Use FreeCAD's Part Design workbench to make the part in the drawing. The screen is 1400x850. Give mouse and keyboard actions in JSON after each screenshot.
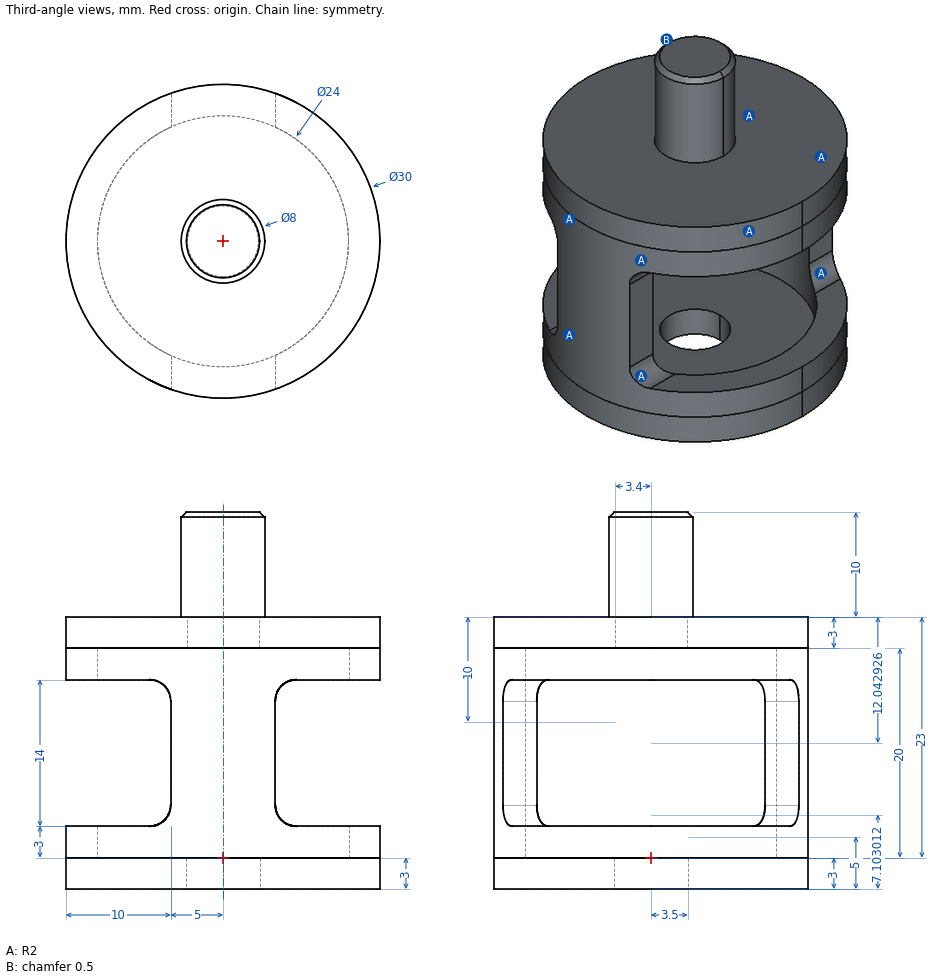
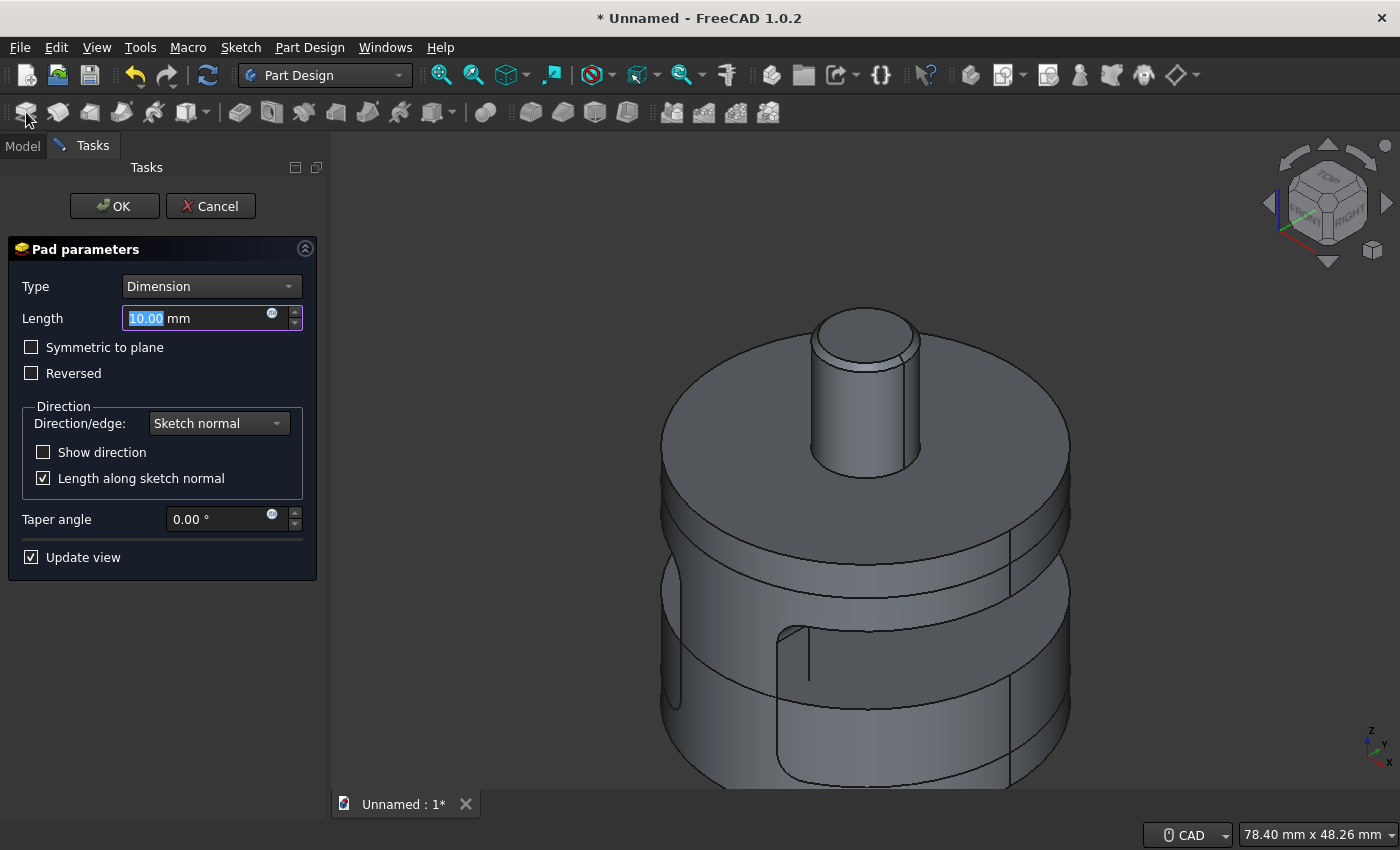
{"action": "type", "text": "3"}
{"action": "key", "text": "Tab"}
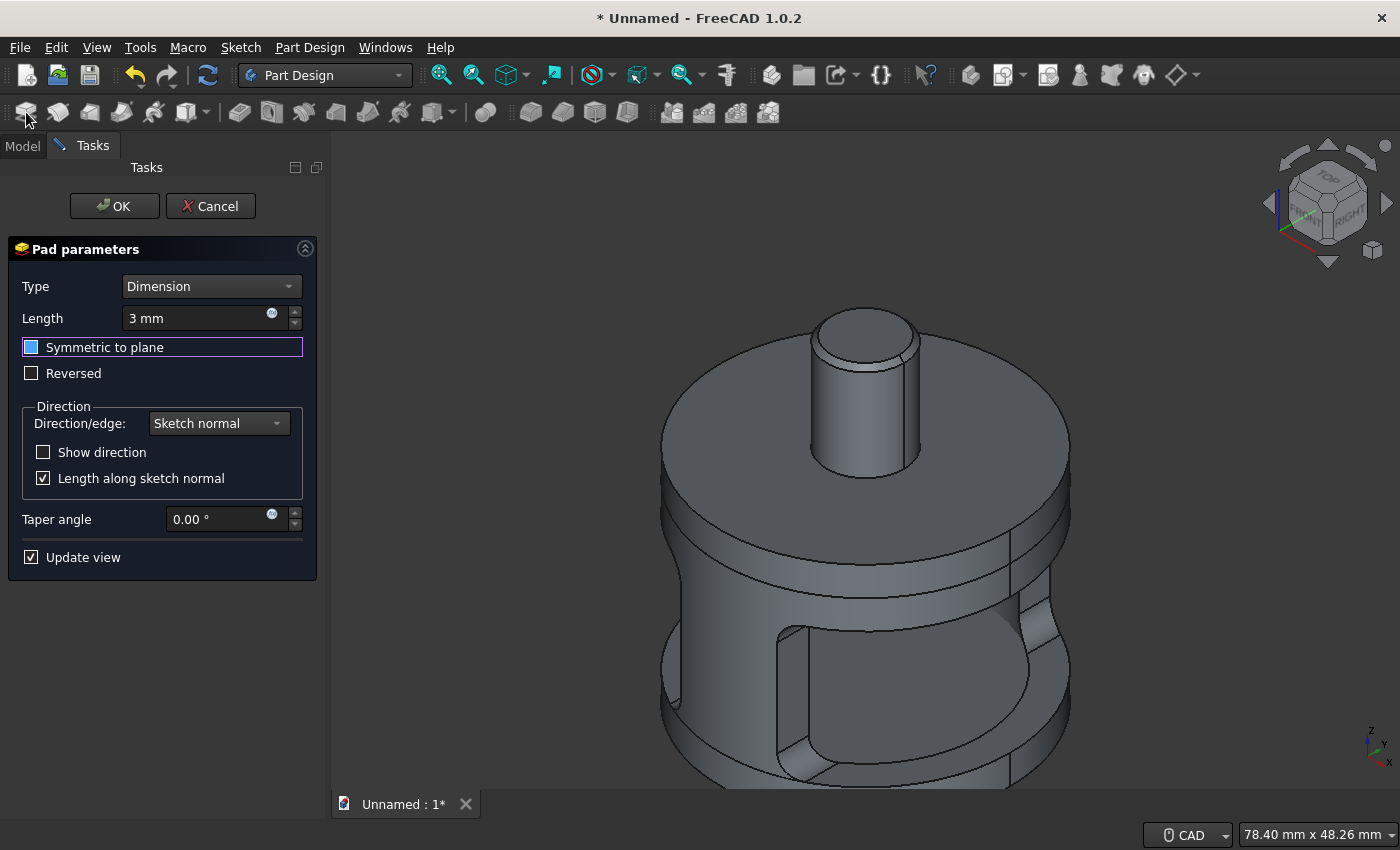
{"action": "left_click", "coordinate": [30, 373]}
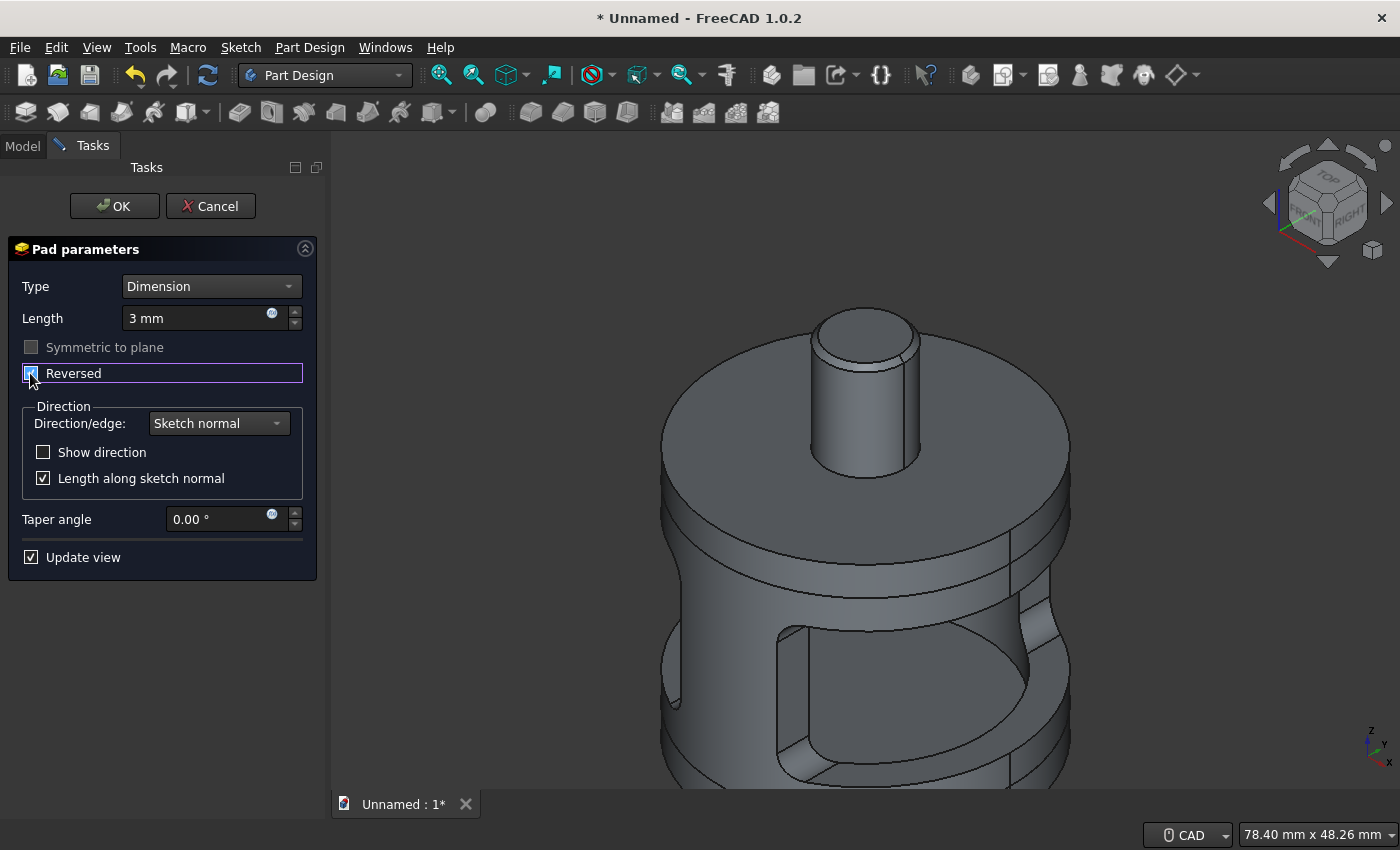
{"action": "left_click", "coordinate": [115, 206]}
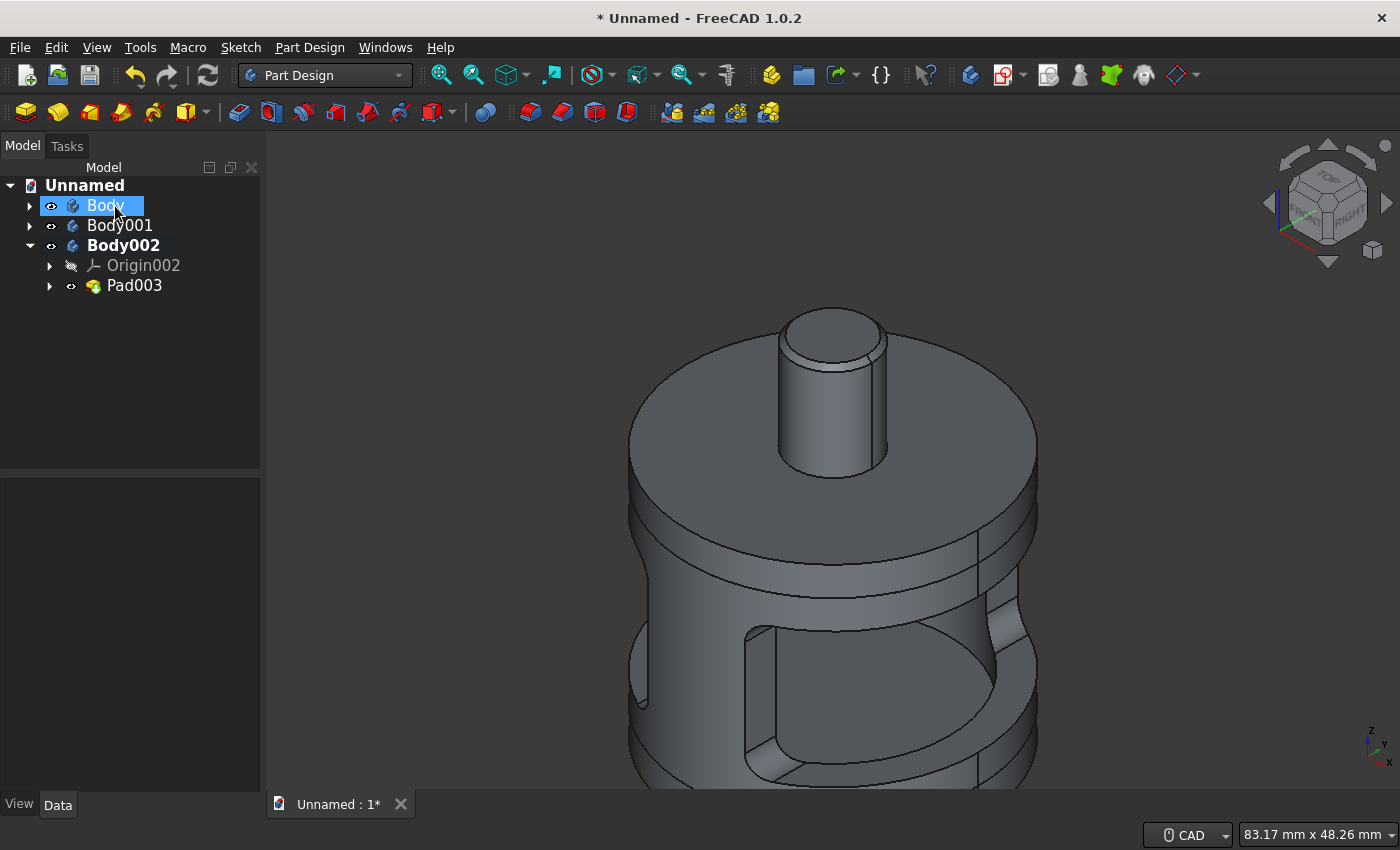
{"action": "left_click", "coordinate": [442, 76]}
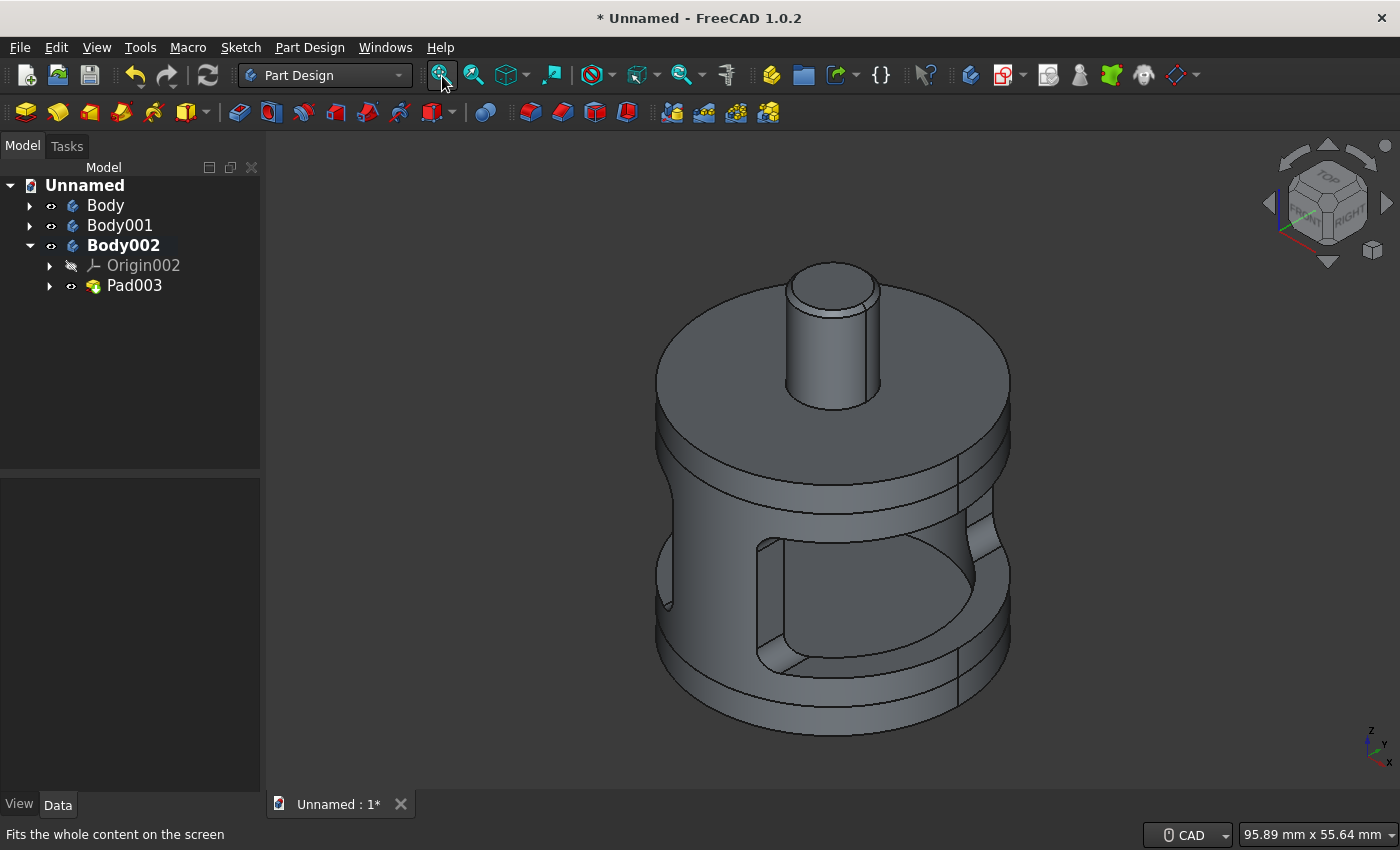
{"action": "left_click", "coordinate": [1004, 76]}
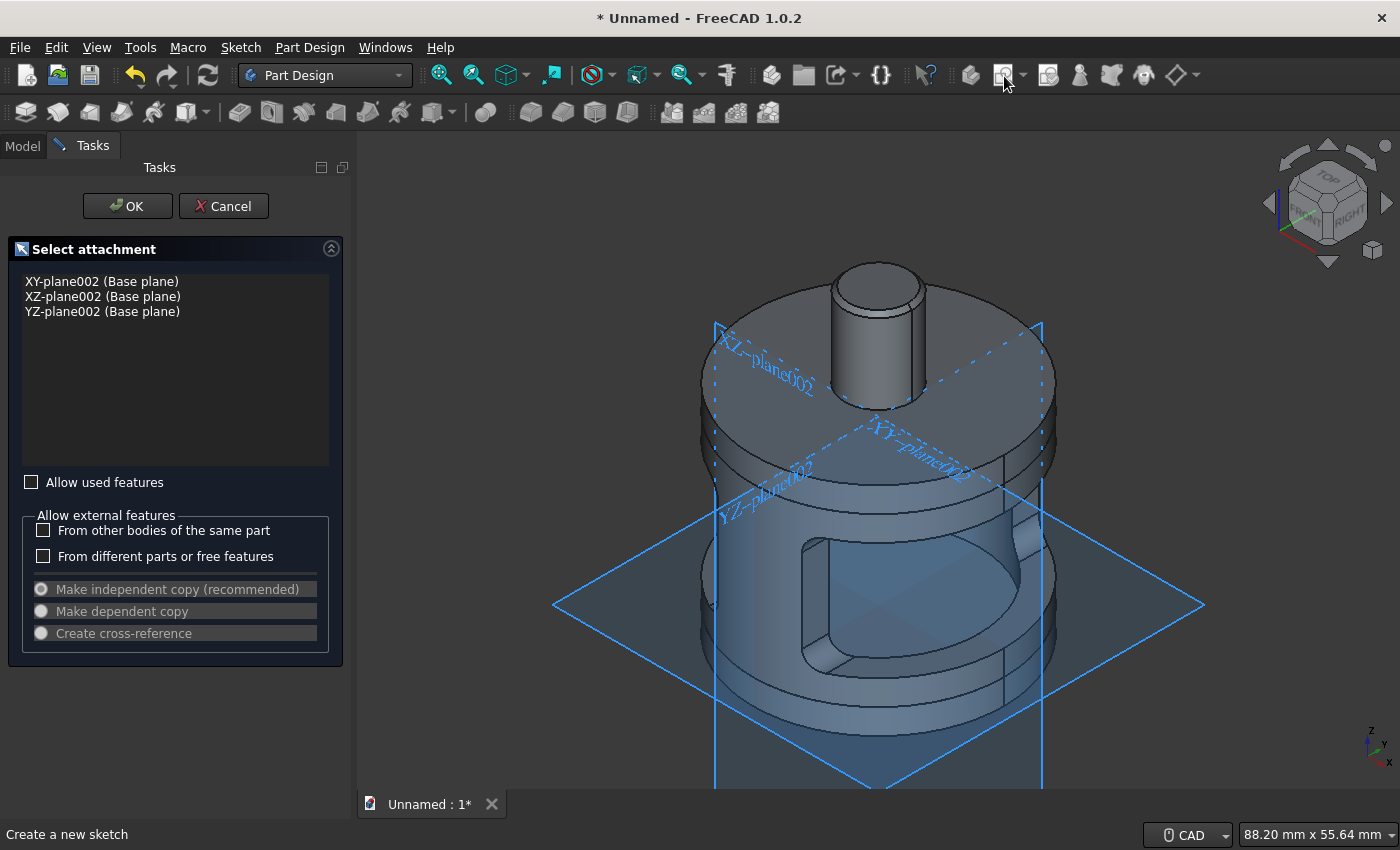
{"action": "left_click", "coordinate": [82, 312]}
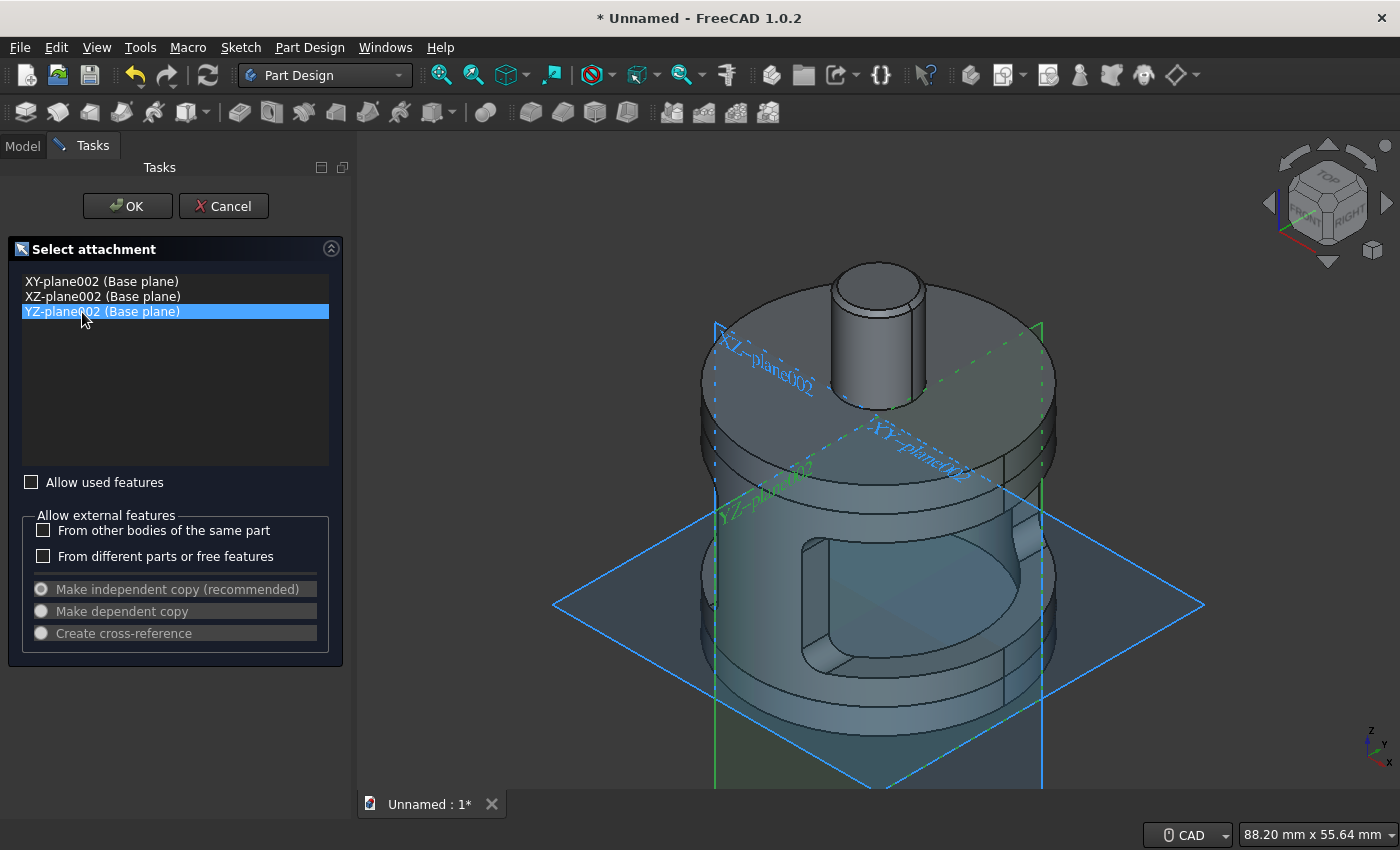
{"action": "left_click", "coordinate": [128, 206]}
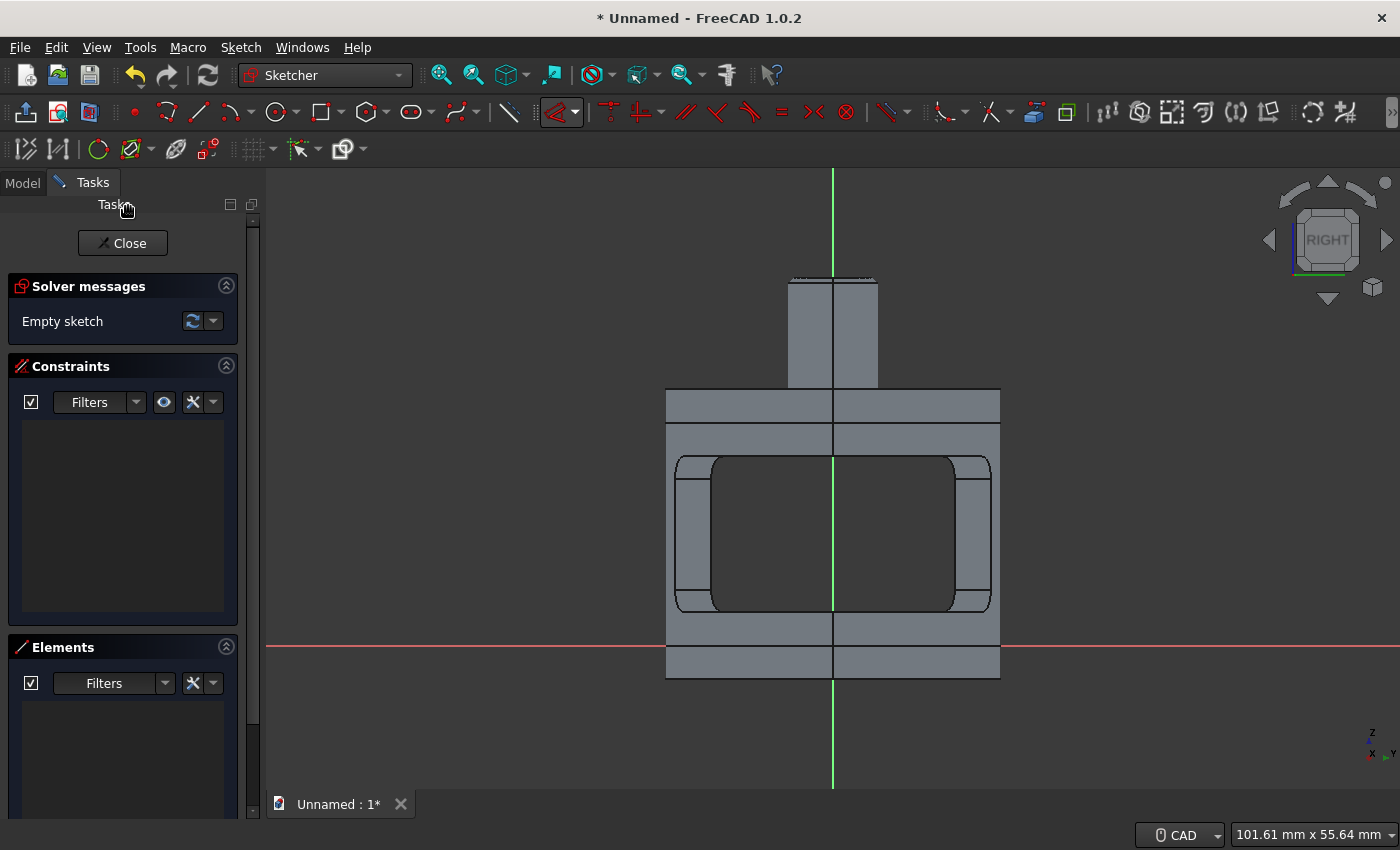
{"action": "left_click", "coordinate": [90, 112]}